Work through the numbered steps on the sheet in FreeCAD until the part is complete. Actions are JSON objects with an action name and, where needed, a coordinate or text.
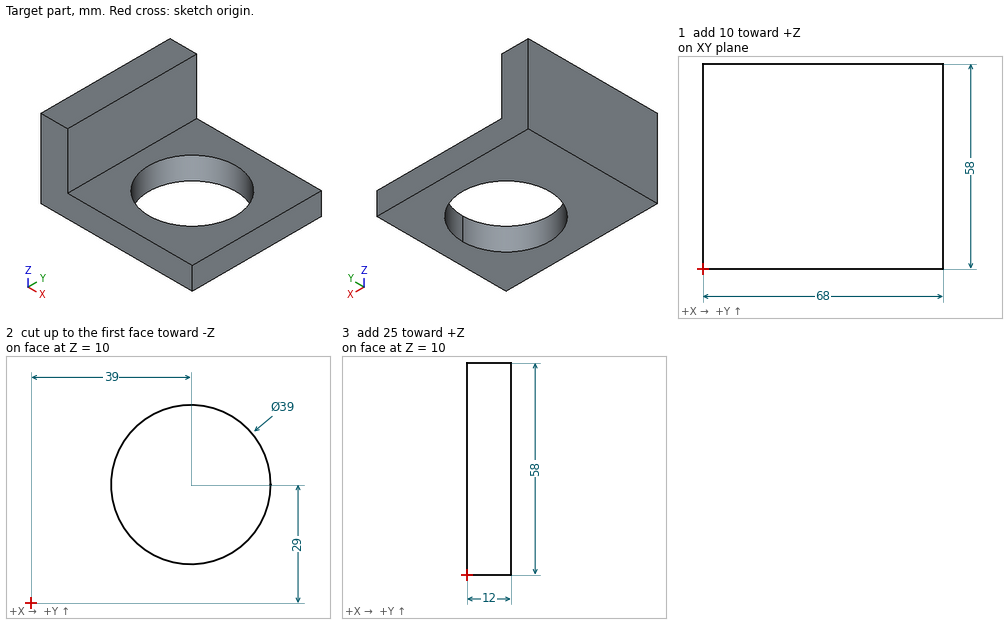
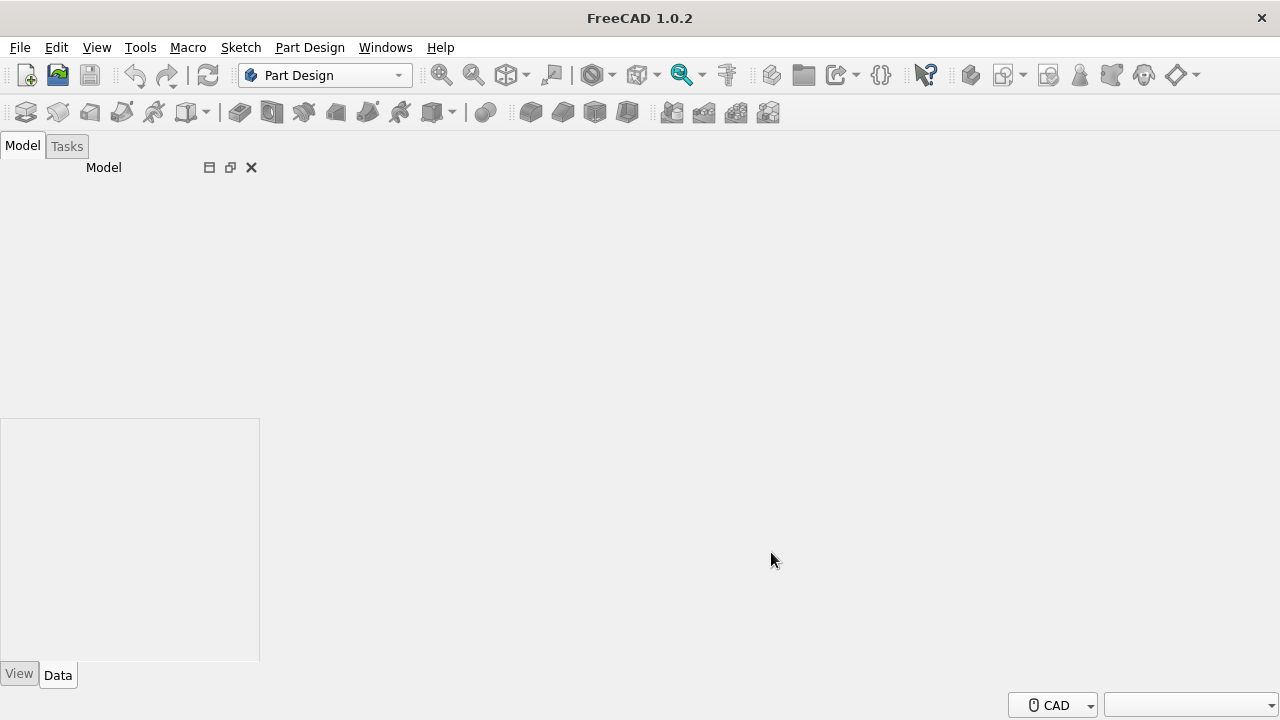
{"action": "key", "text": "ctrl+n"}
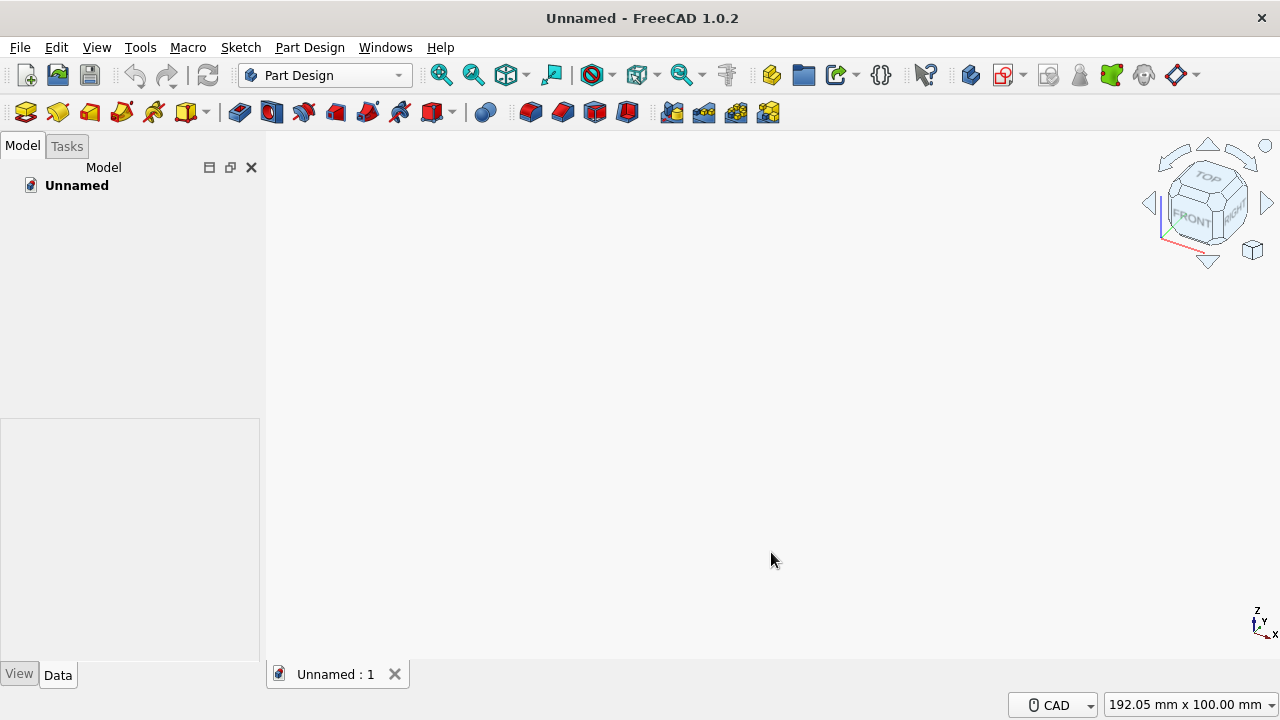
{"action": "left_click", "coordinate": [1004, 76]}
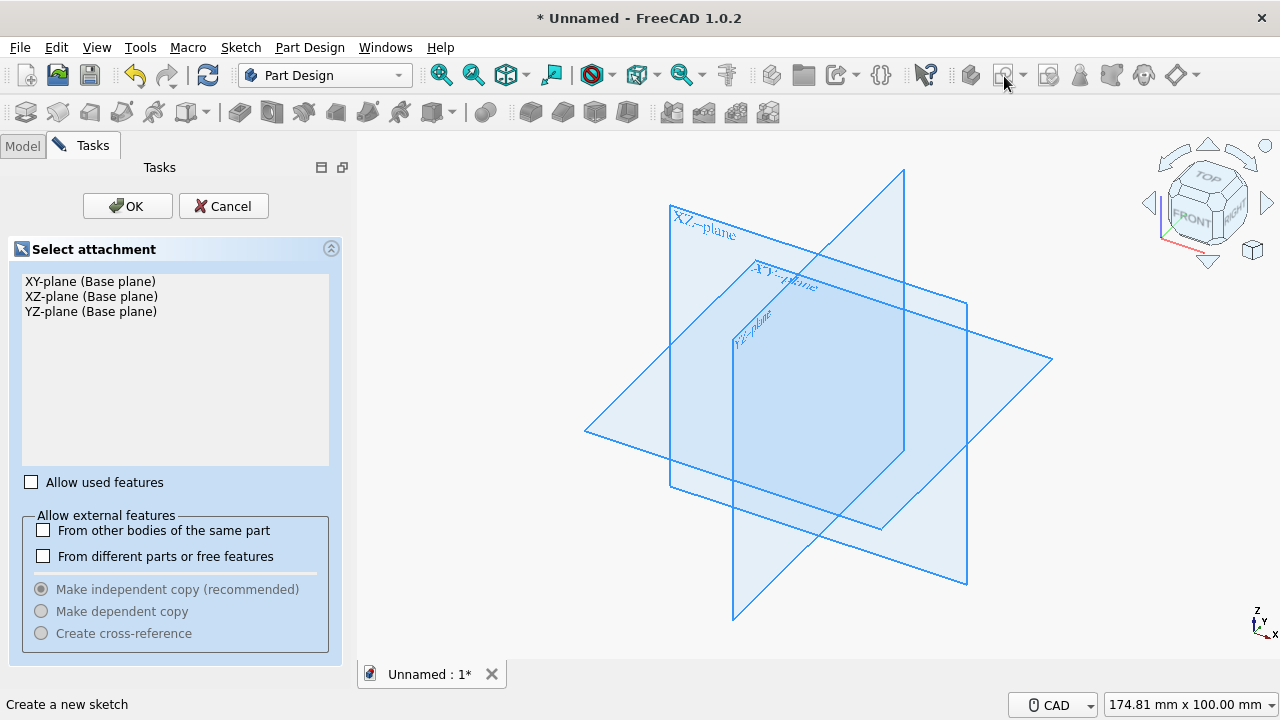
{"action": "left_click", "coordinate": [82, 282]}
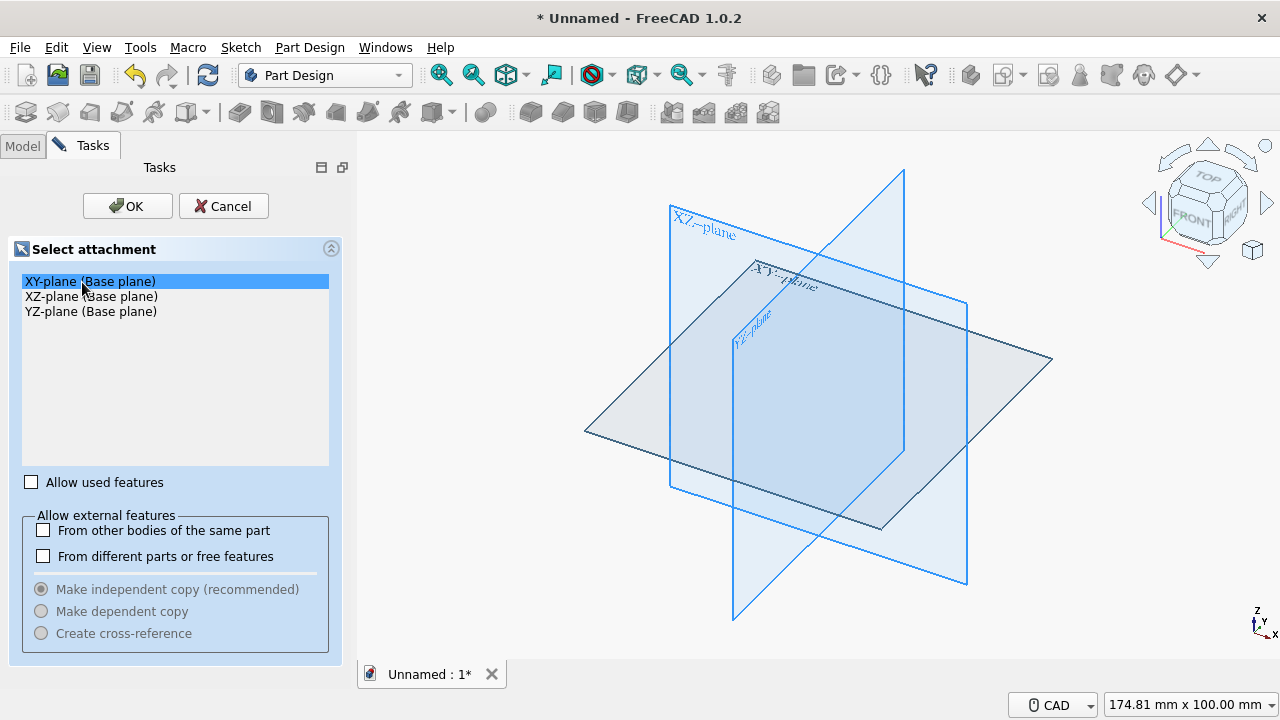
{"action": "left_click", "coordinate": [128, 206]}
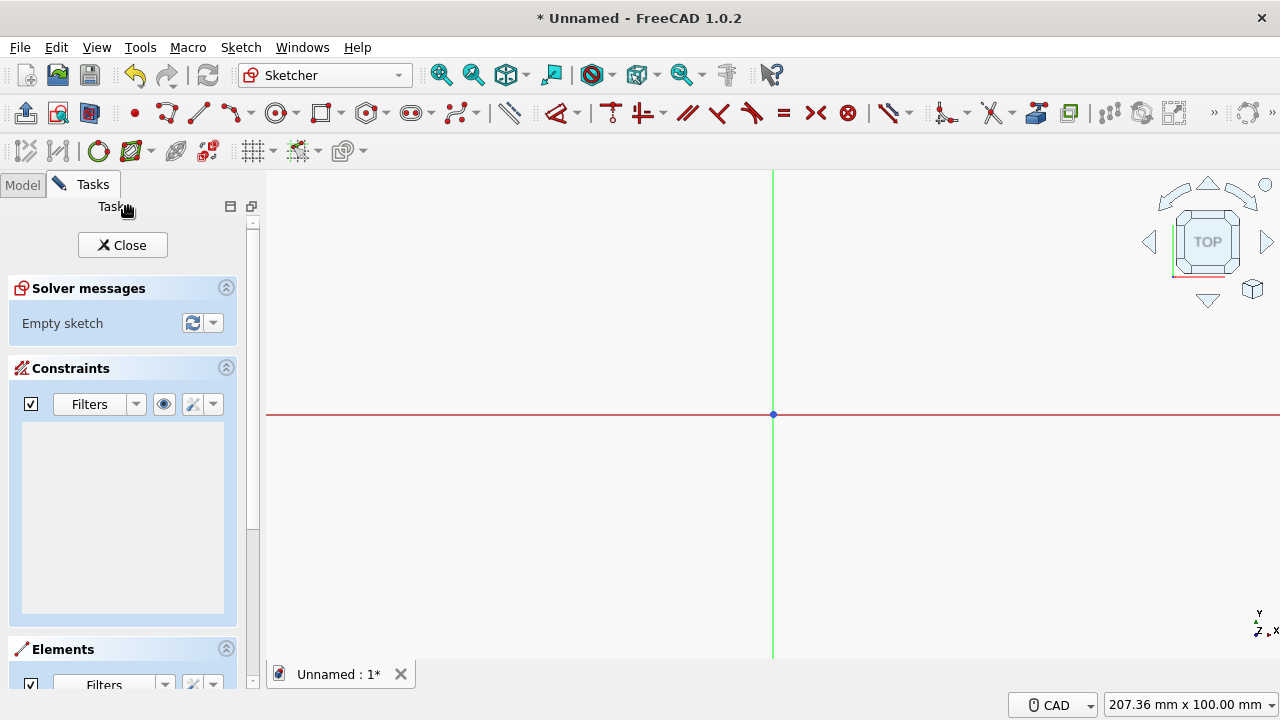
{"action": "scroll", "coordinate": [294, 631], "scroll_direction": "down", "scroll_amount": 2}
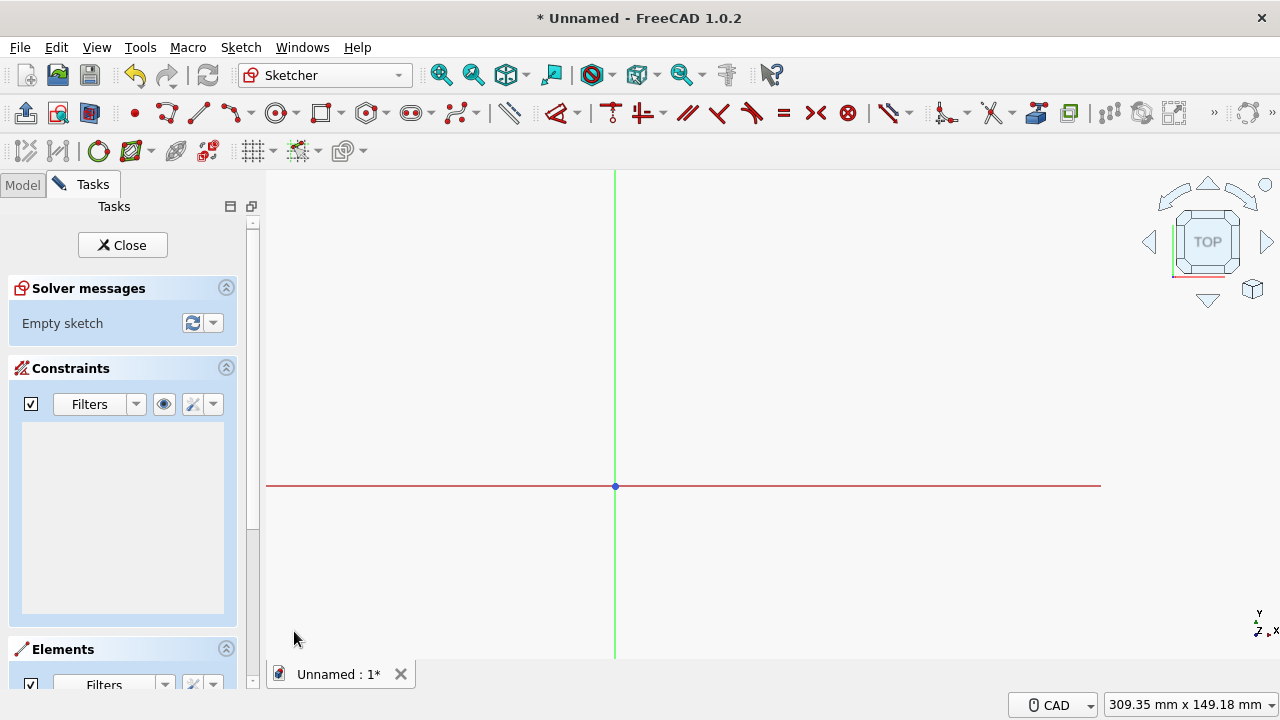
{"action": "scroll", "coordinate": [771, 344], "scroll_direction": "up", "scroll_amount": 2}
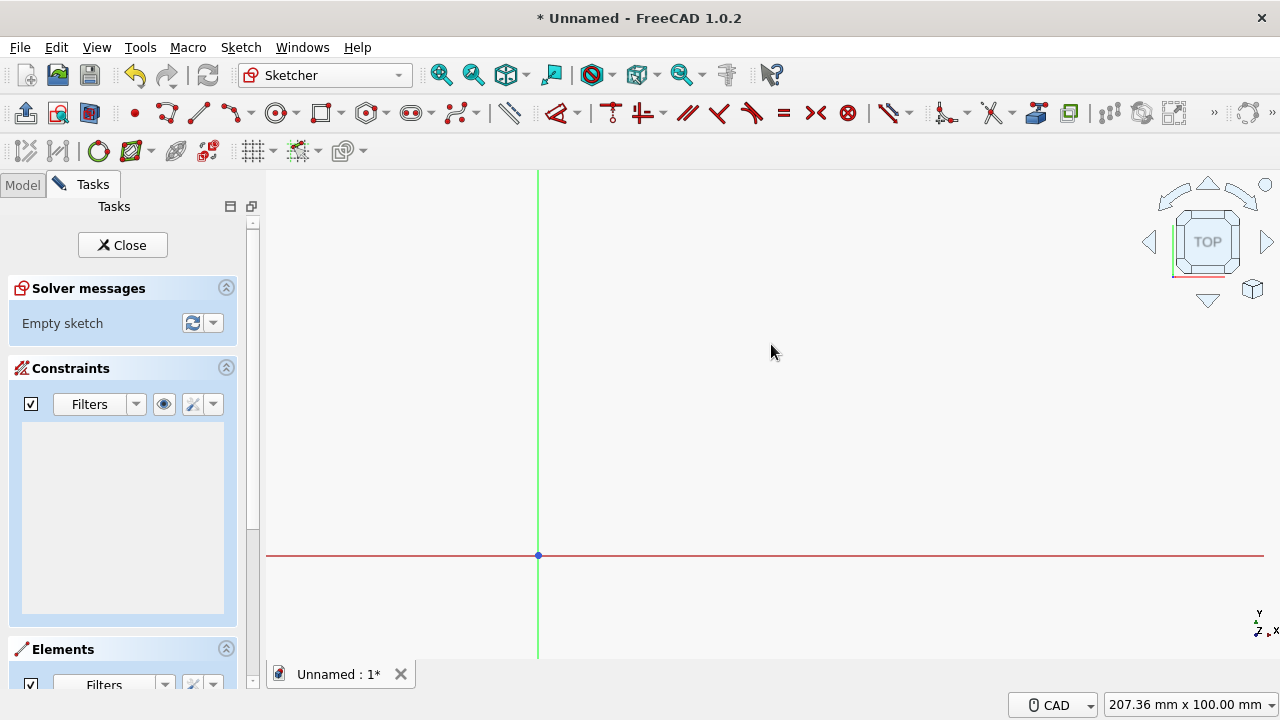
{"action": "left_click", "coordinate": [322, 114]}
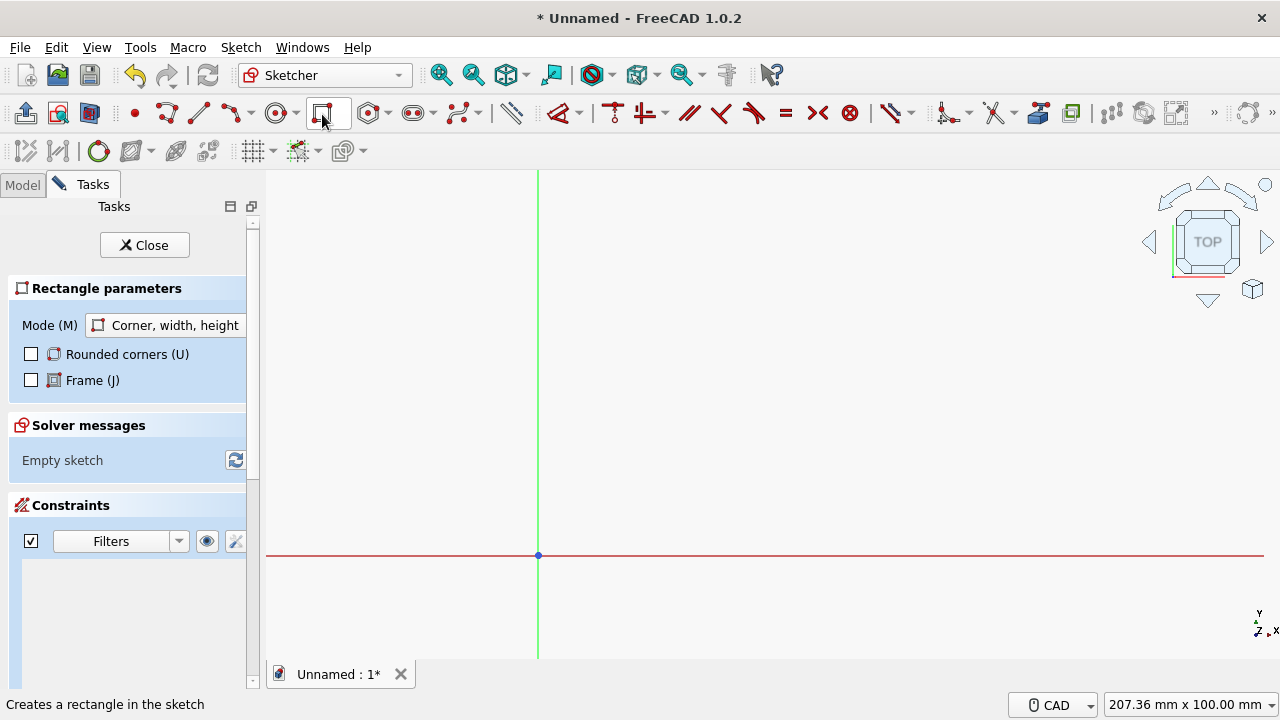
{"action": "left_click", "coordinate": [538, 556]}
{"action": "left_click", "coordinate": [871, 272]}
{"action": "key", "text": "Escape"}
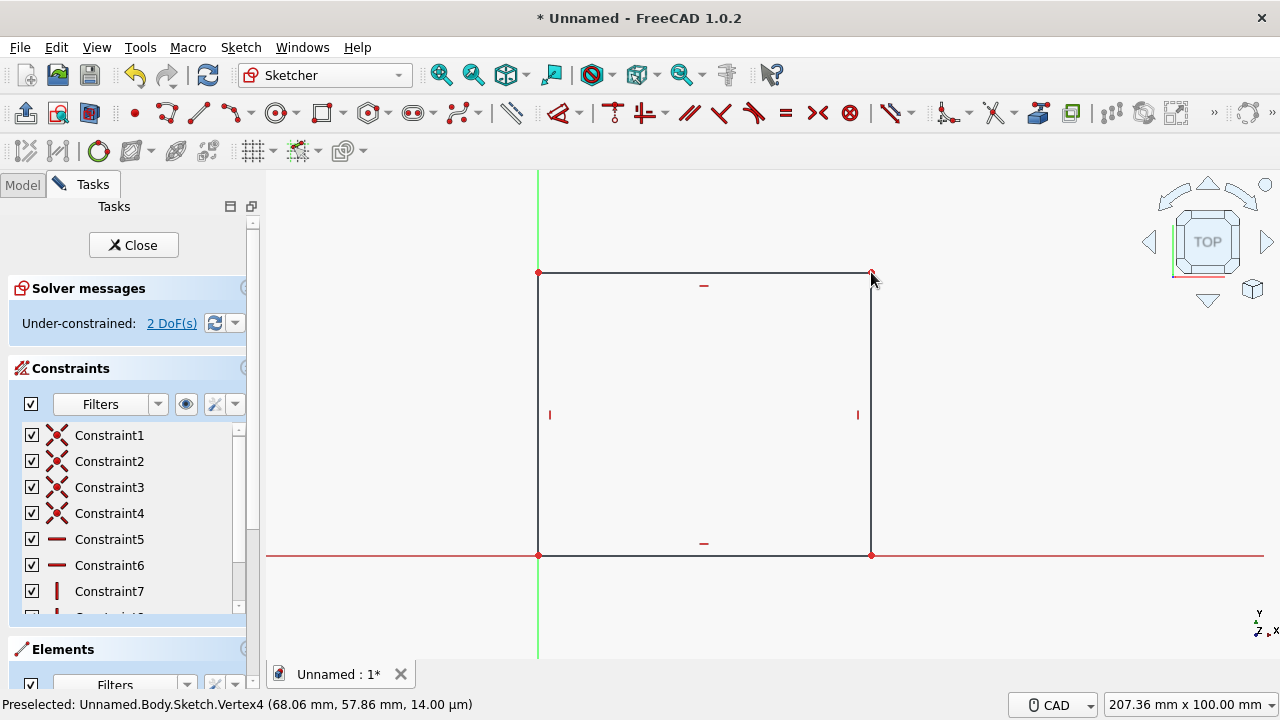
{"action": "left_click", "coordinate": [638, 556]}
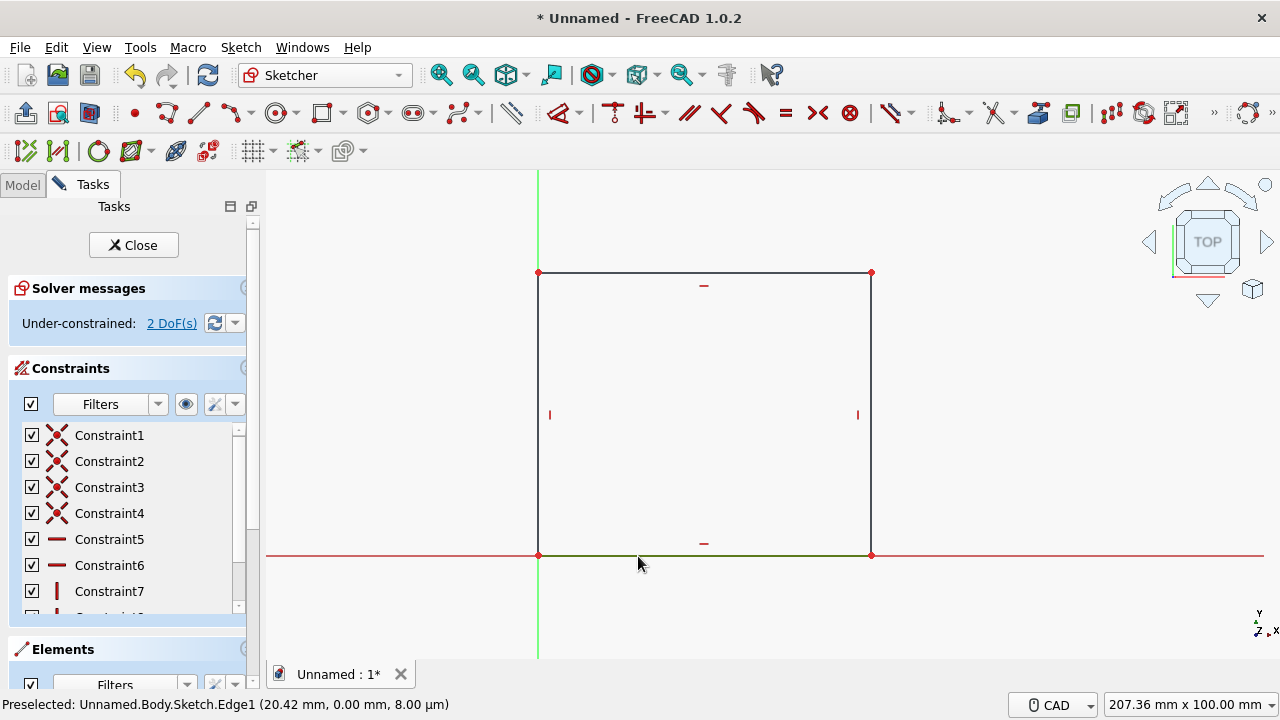
{"action": "key", "text": "l"}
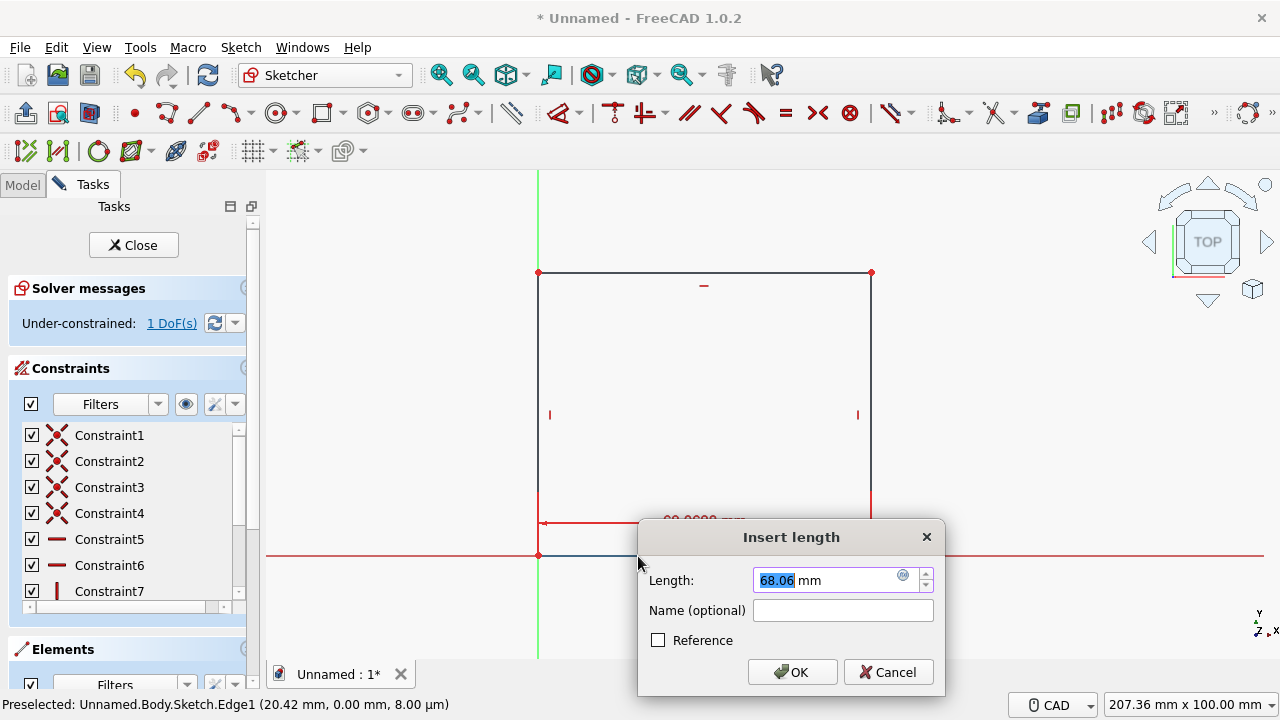
{"action": "type", "text": "68"}
{"action": "key", "text": "Return"}